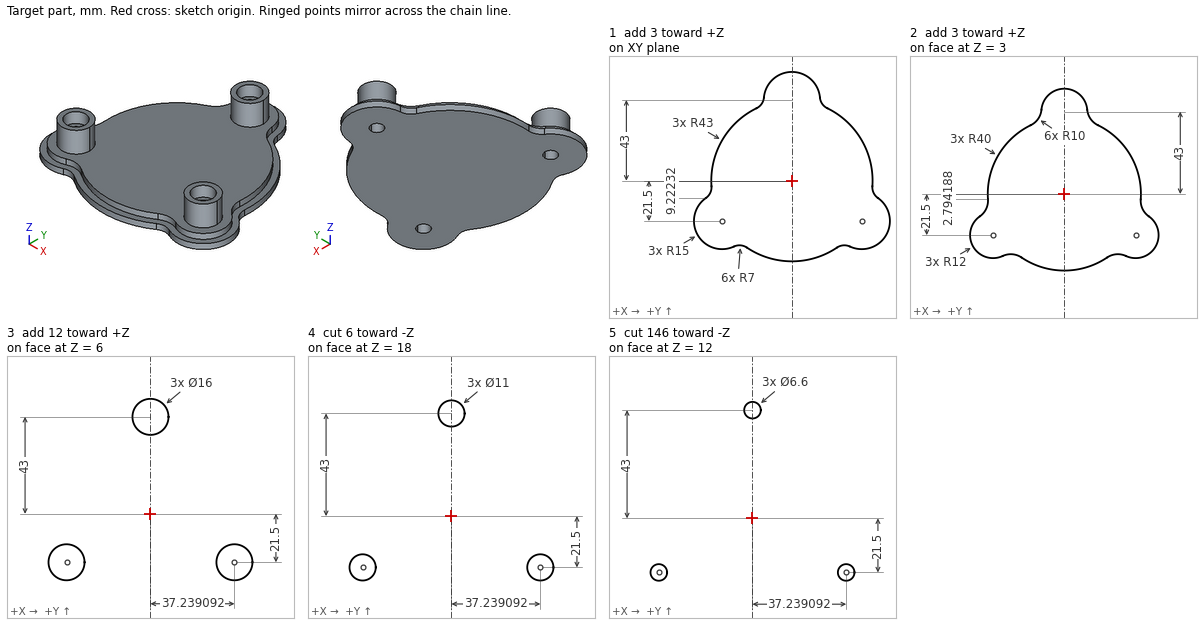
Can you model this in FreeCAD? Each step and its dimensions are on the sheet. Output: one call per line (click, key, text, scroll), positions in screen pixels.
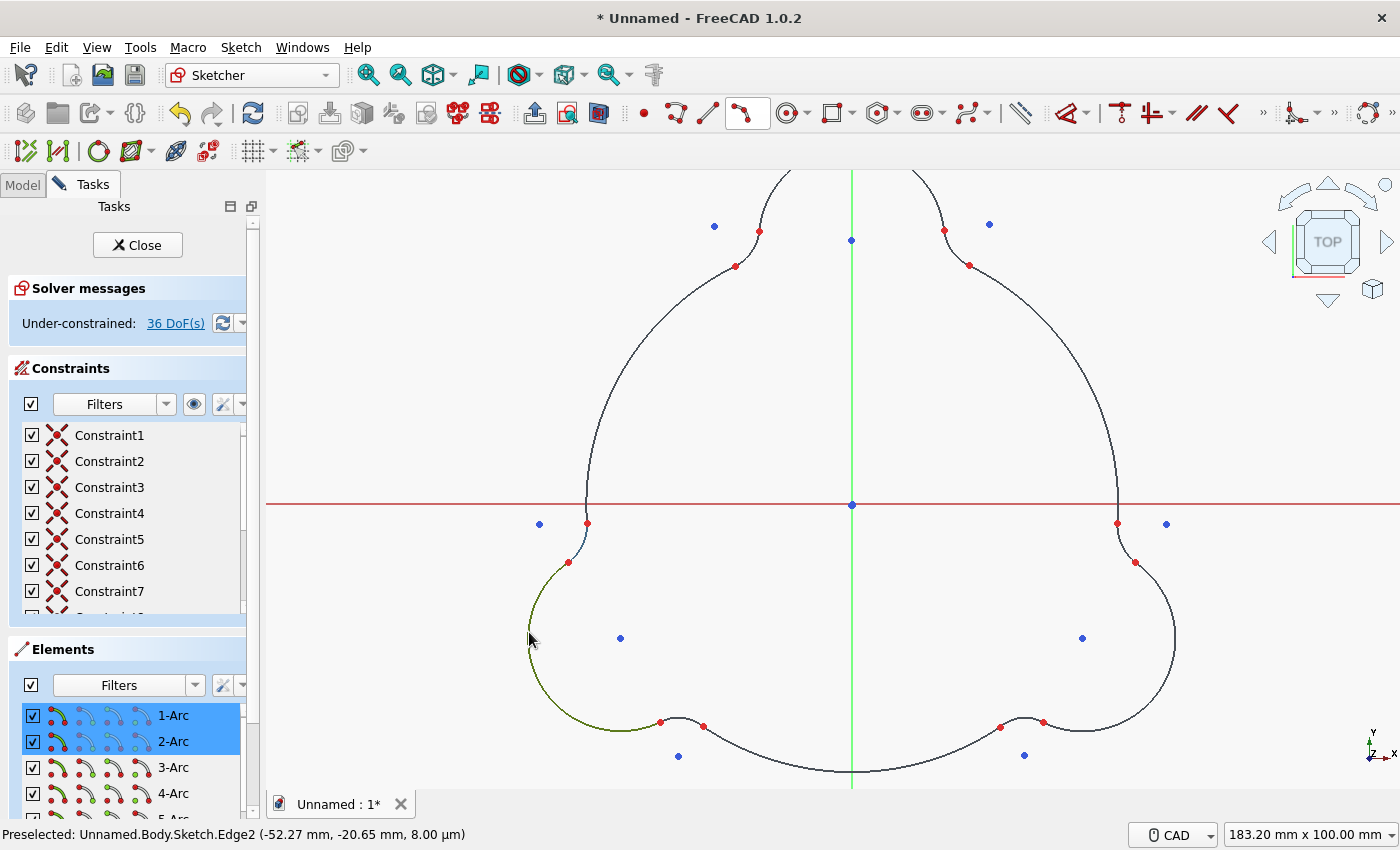
key(t)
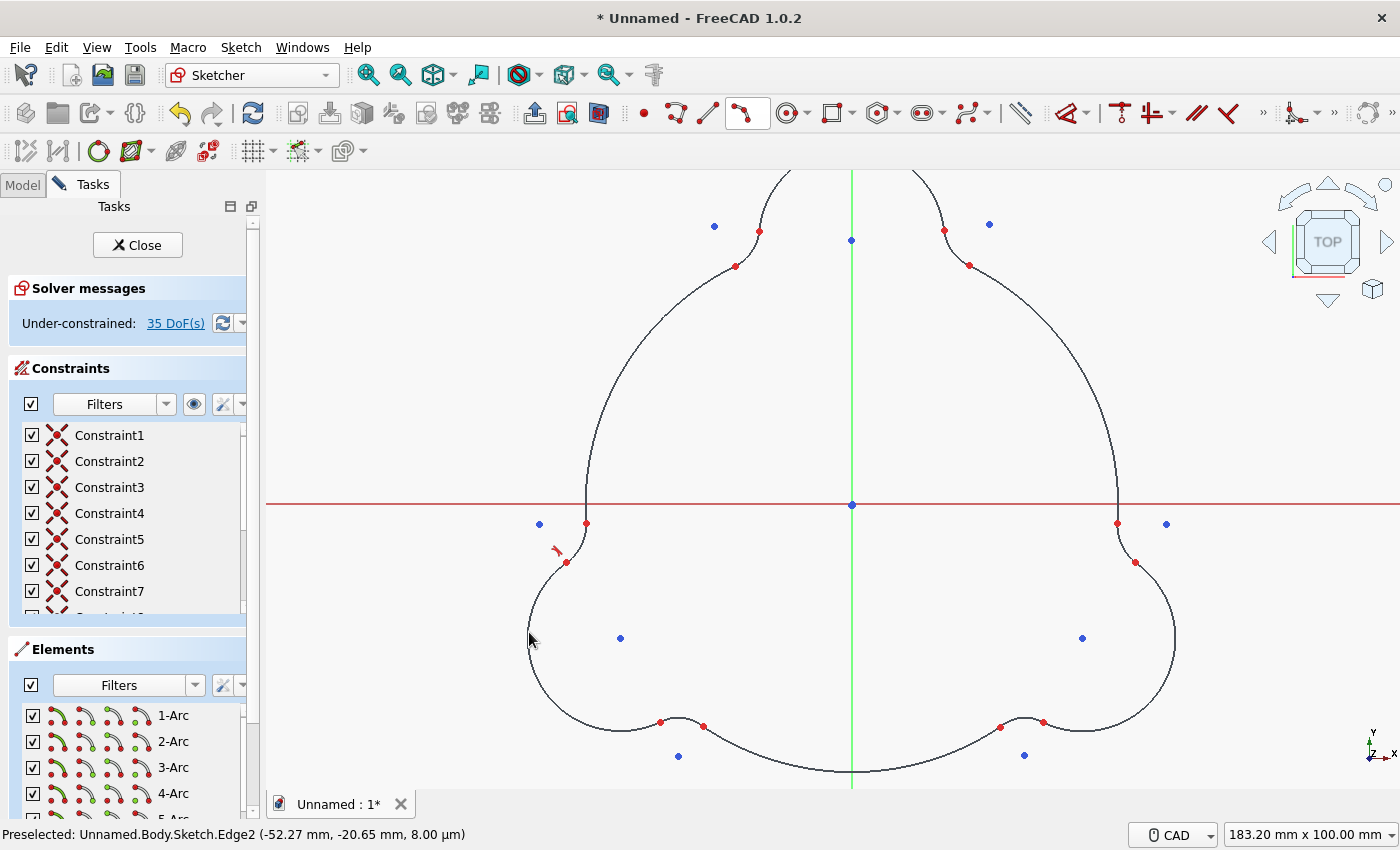
click(576, 553)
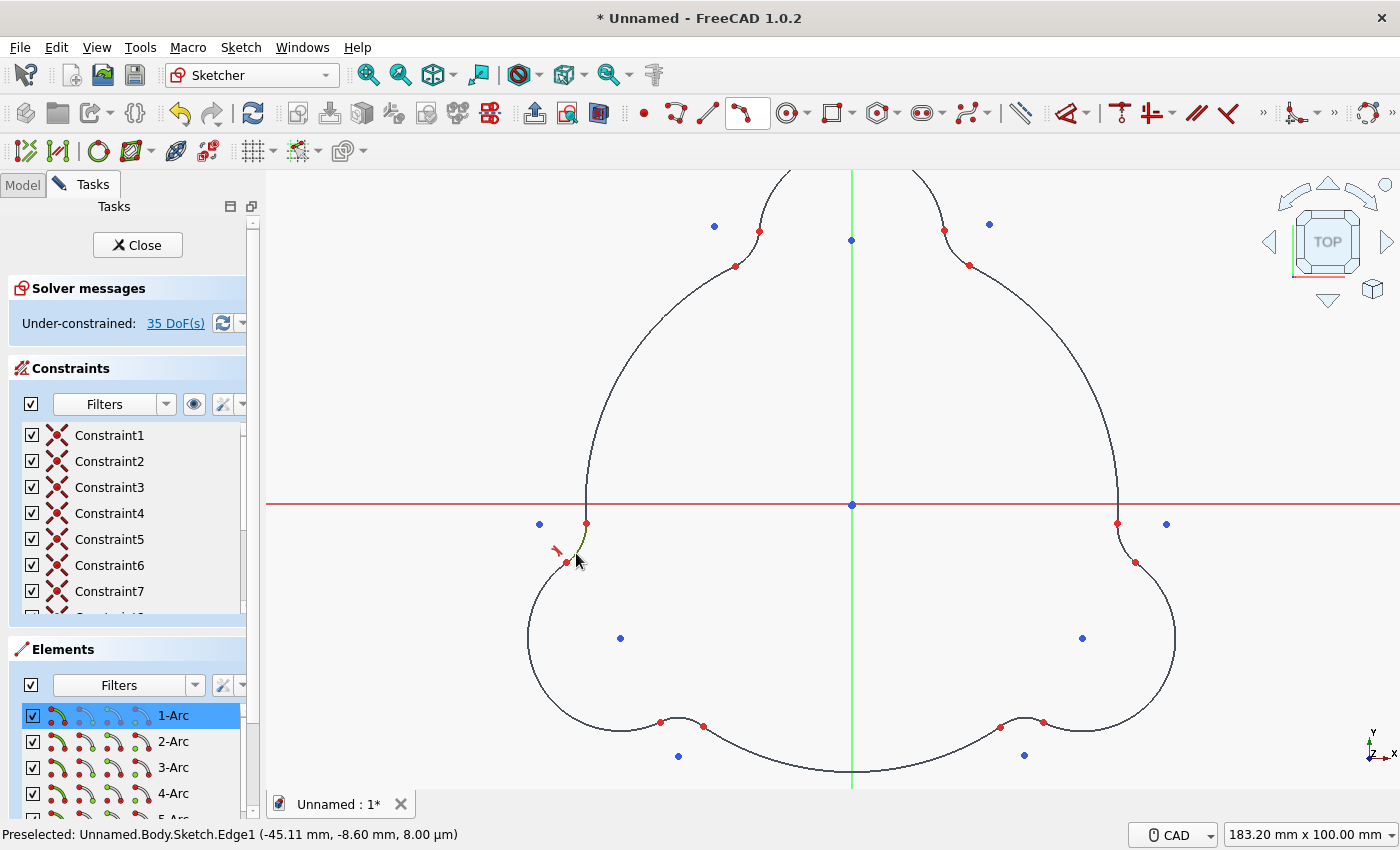
click(659, 322)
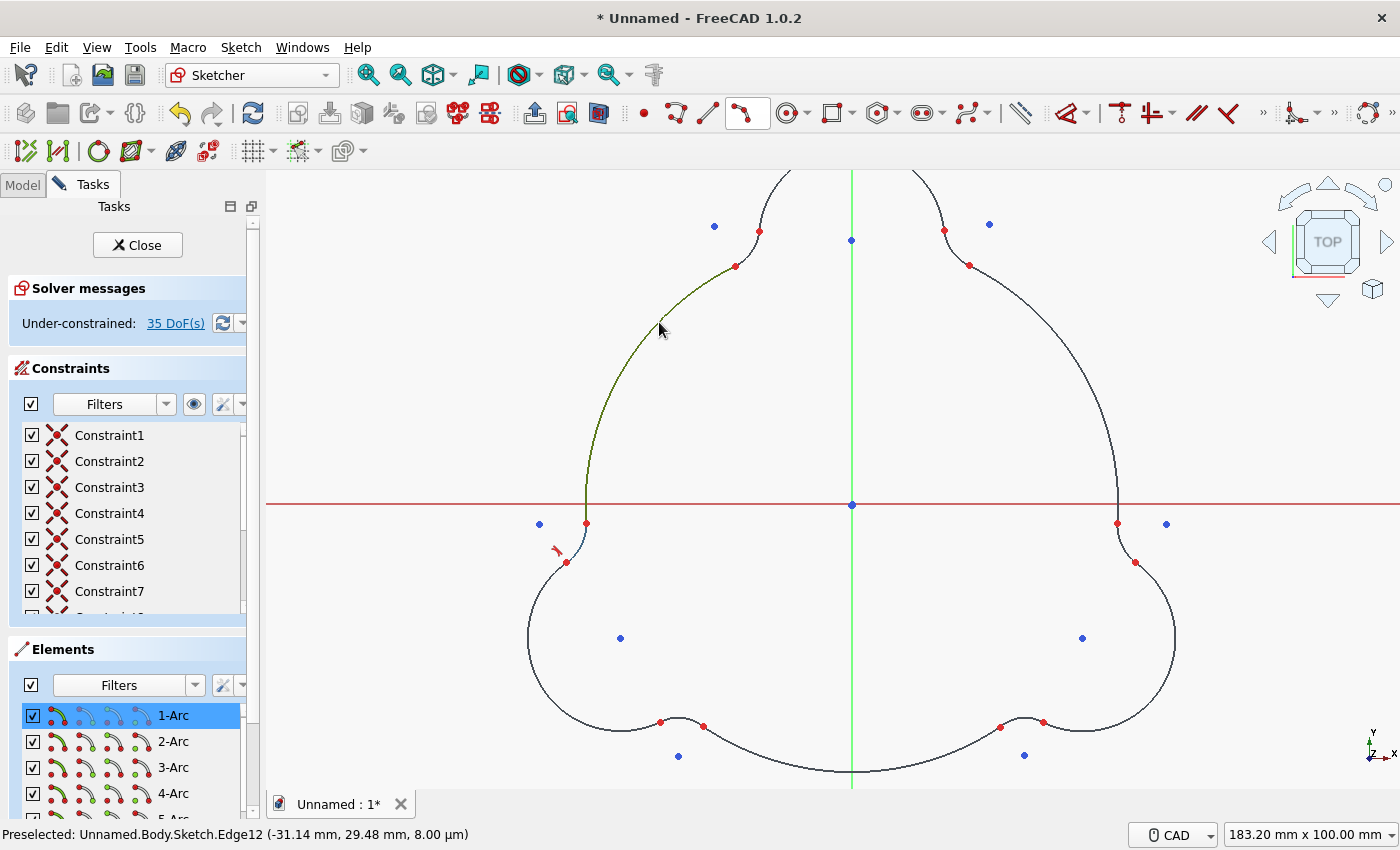
key(t)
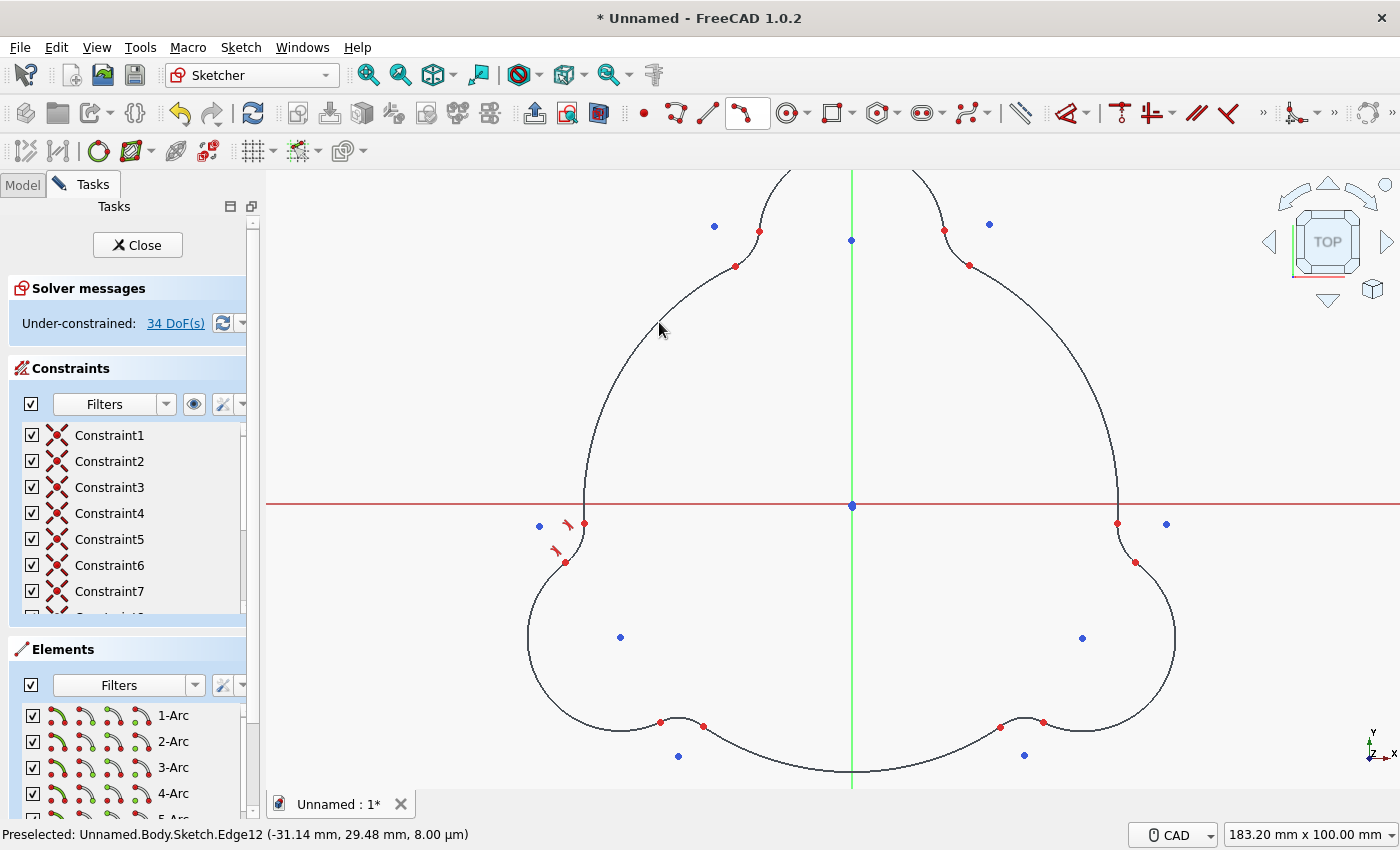
click(528, 633)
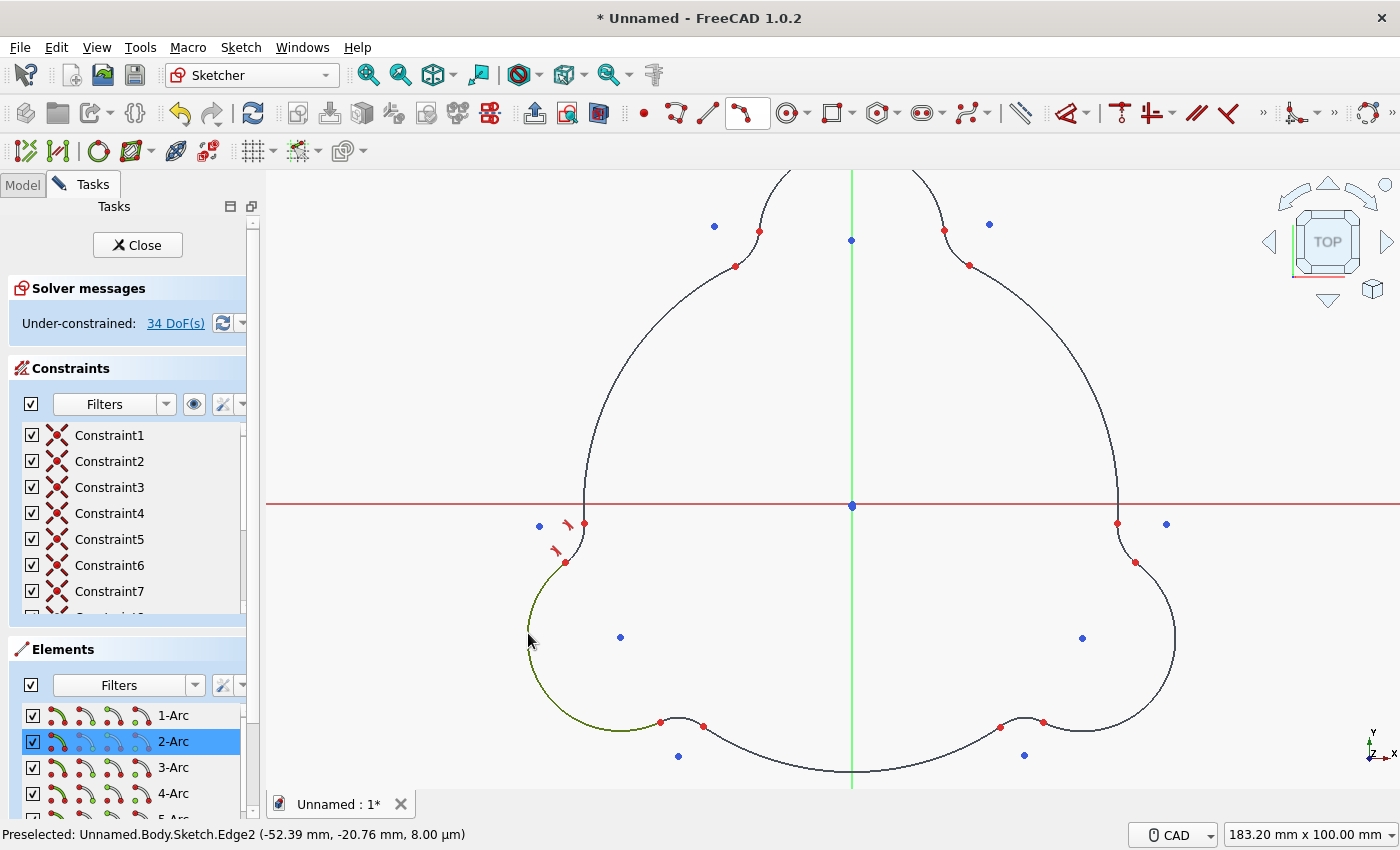
click(691, 720)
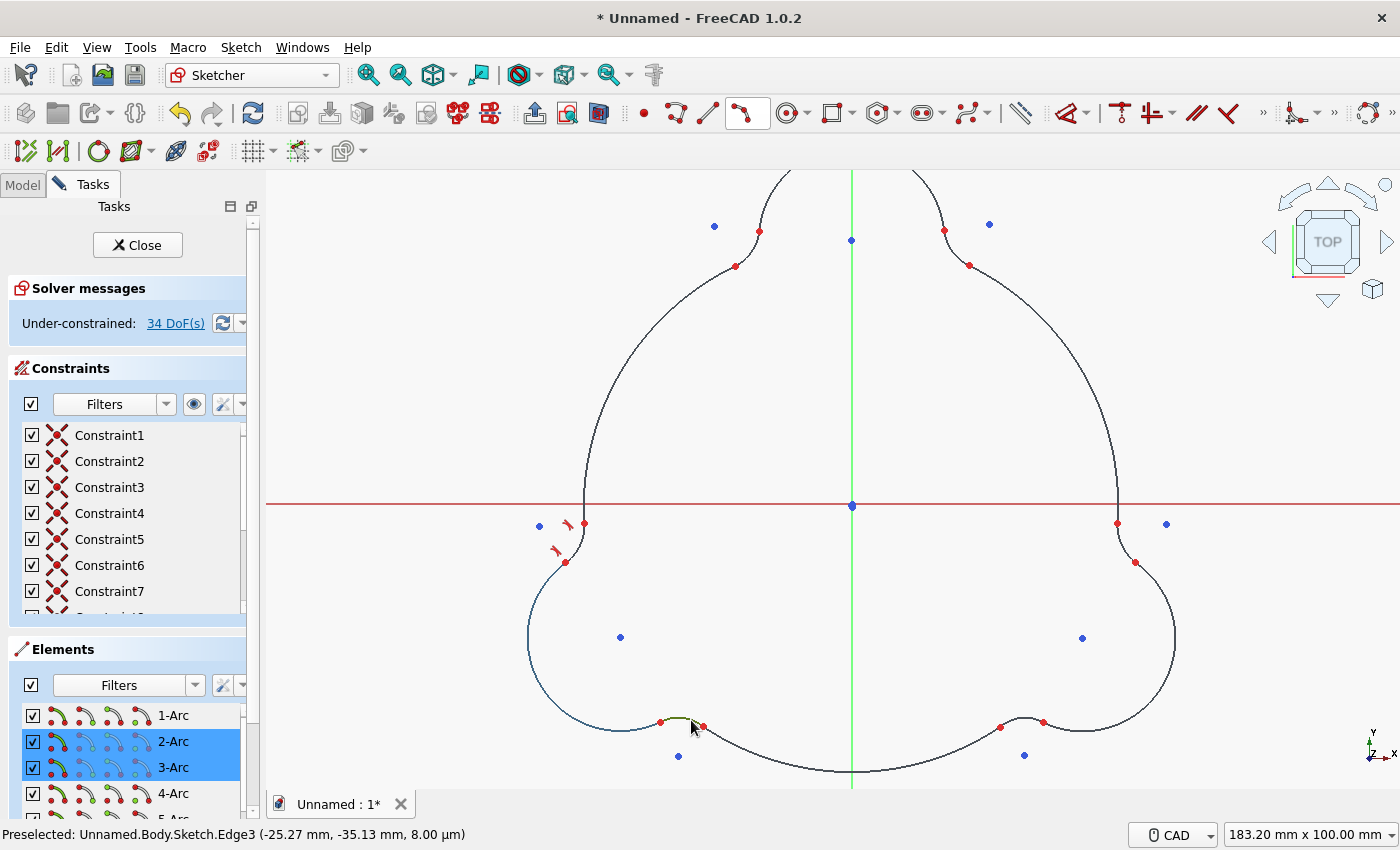
key(t)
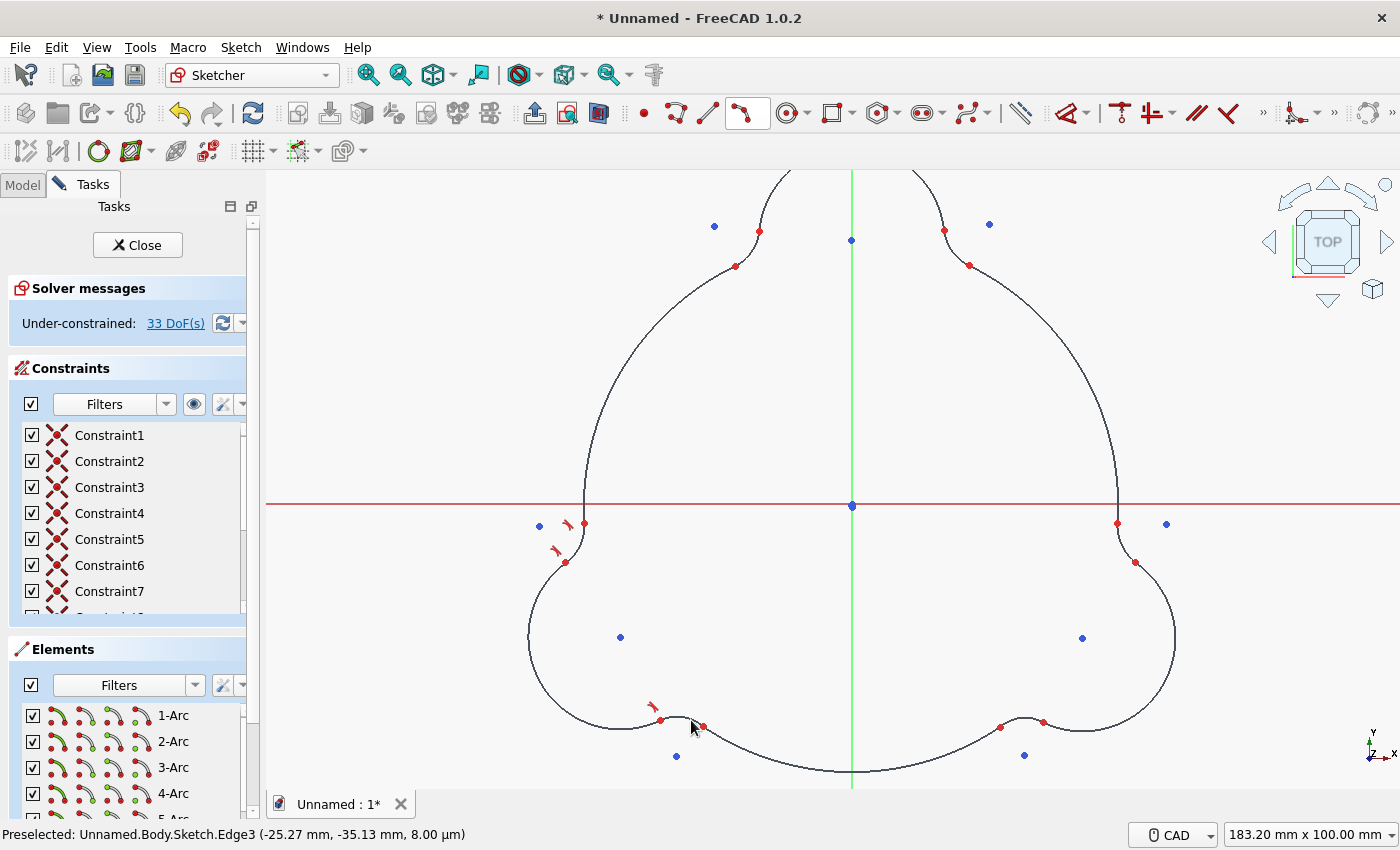
click(692, 720)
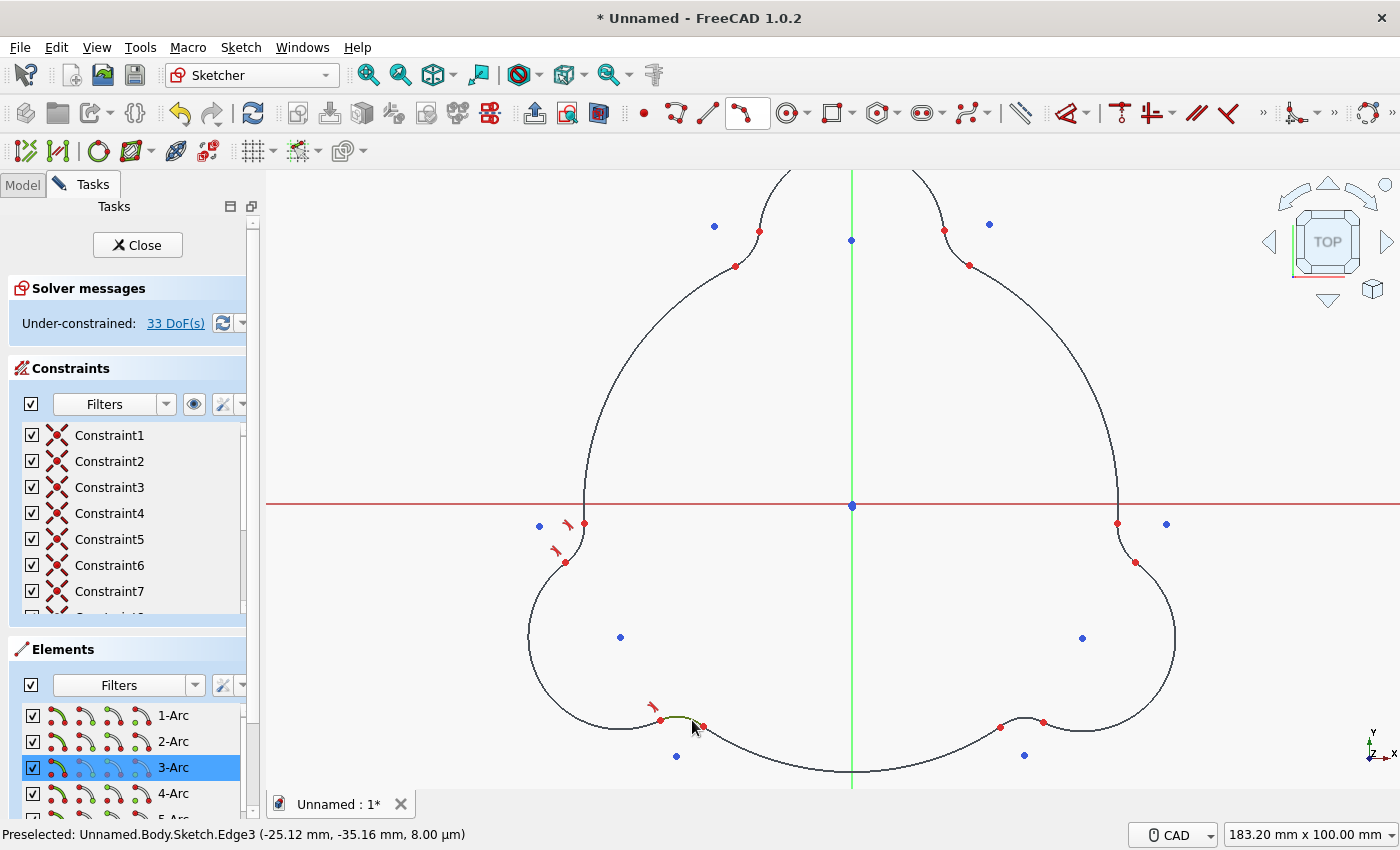
click(759, 755)